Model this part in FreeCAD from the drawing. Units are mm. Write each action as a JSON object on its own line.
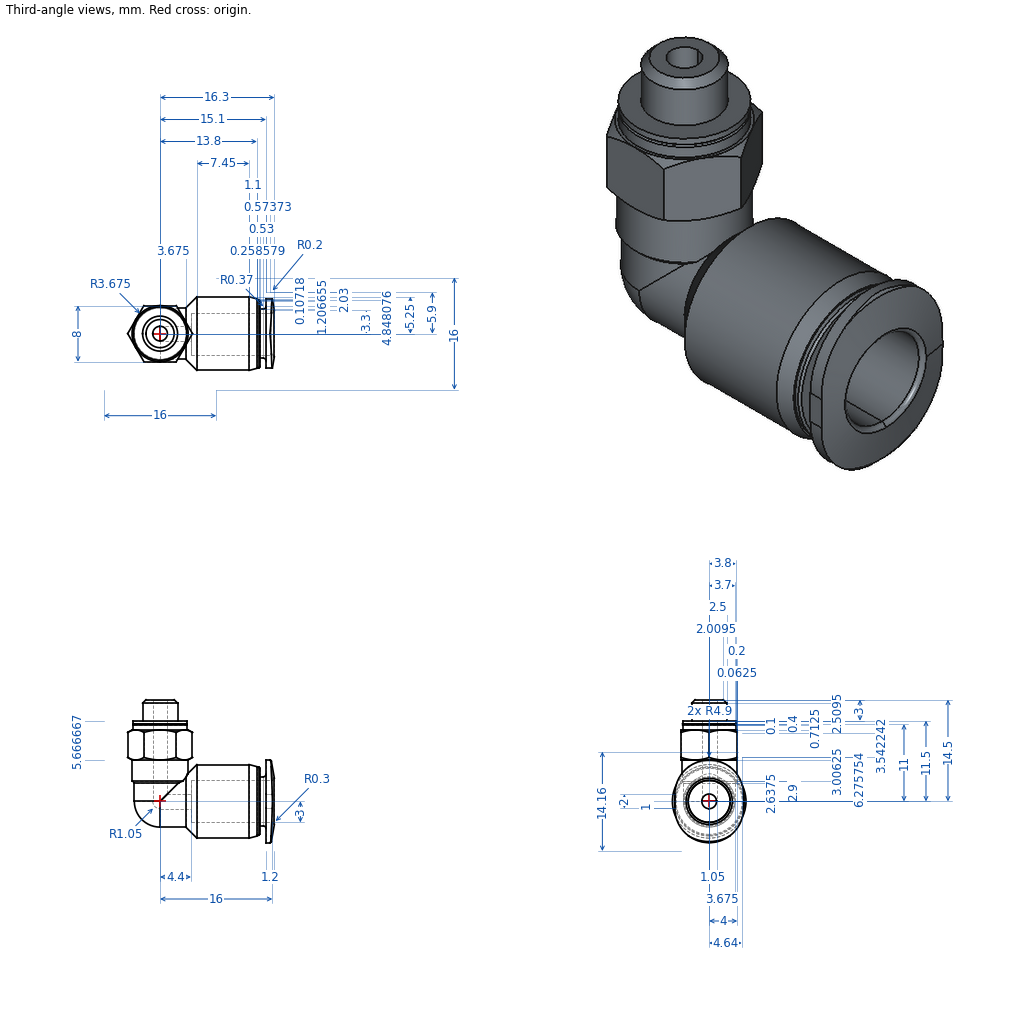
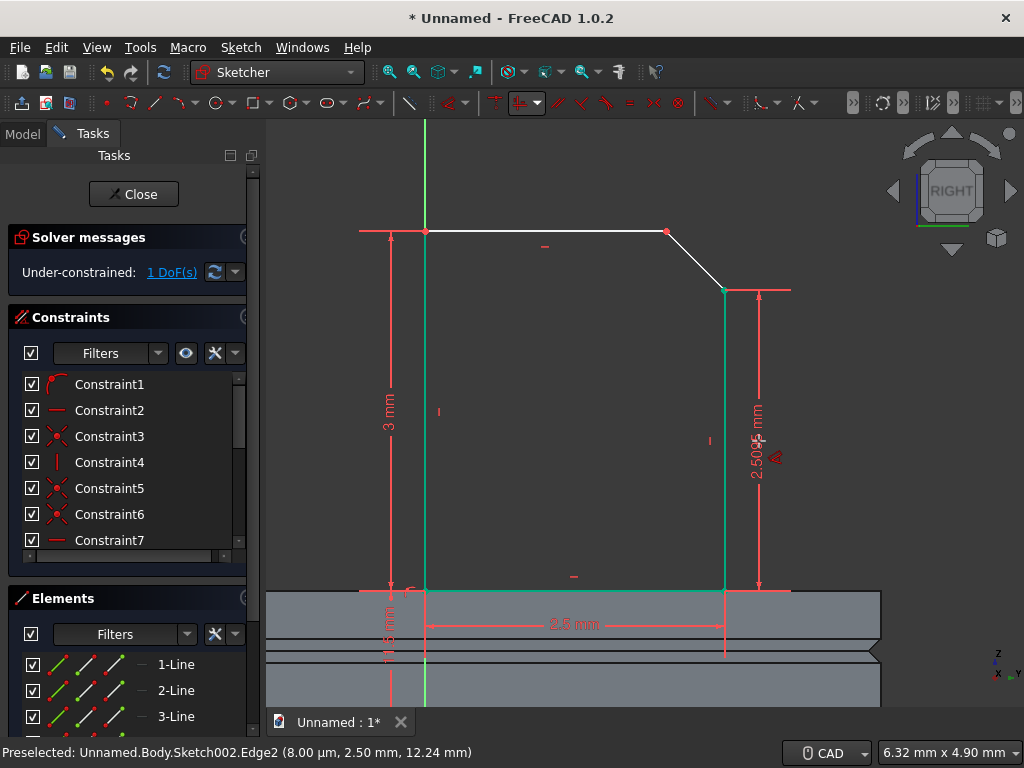
{"action": "left_click", "coordinate": [594, 231]}
{"action": "left_click", "coordinate": [546, 197]}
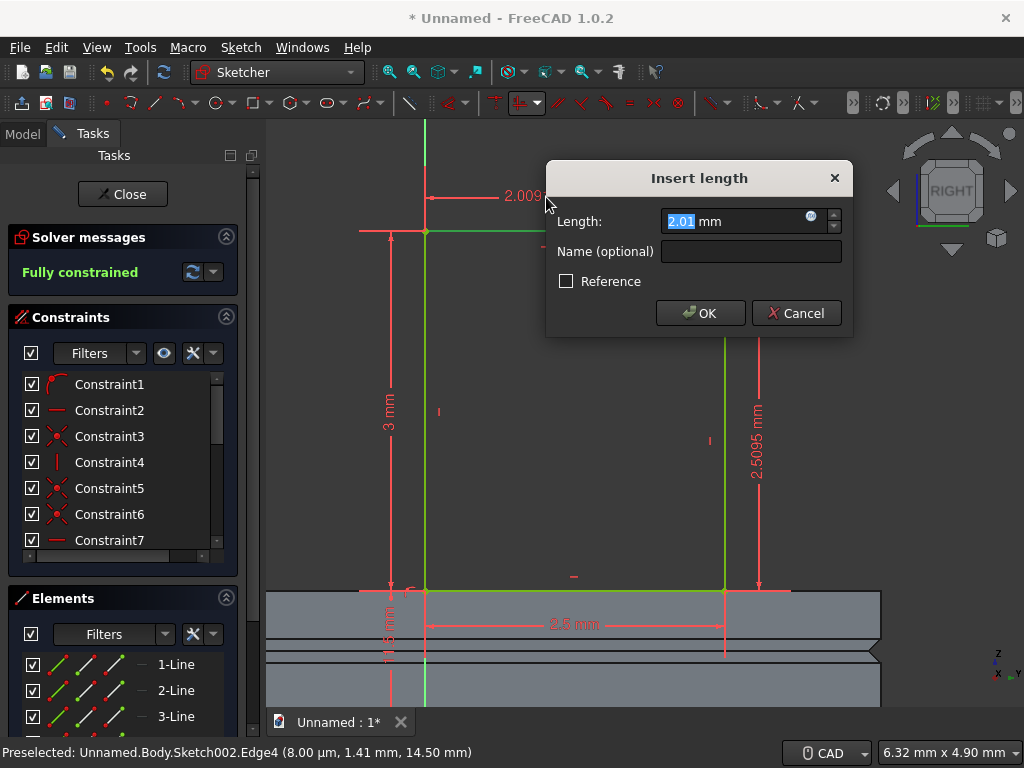
{"action": "type", "text": "2.0095"}
{"action": "key", "text": "Return"}
{"action": "key", "text": "Escape"}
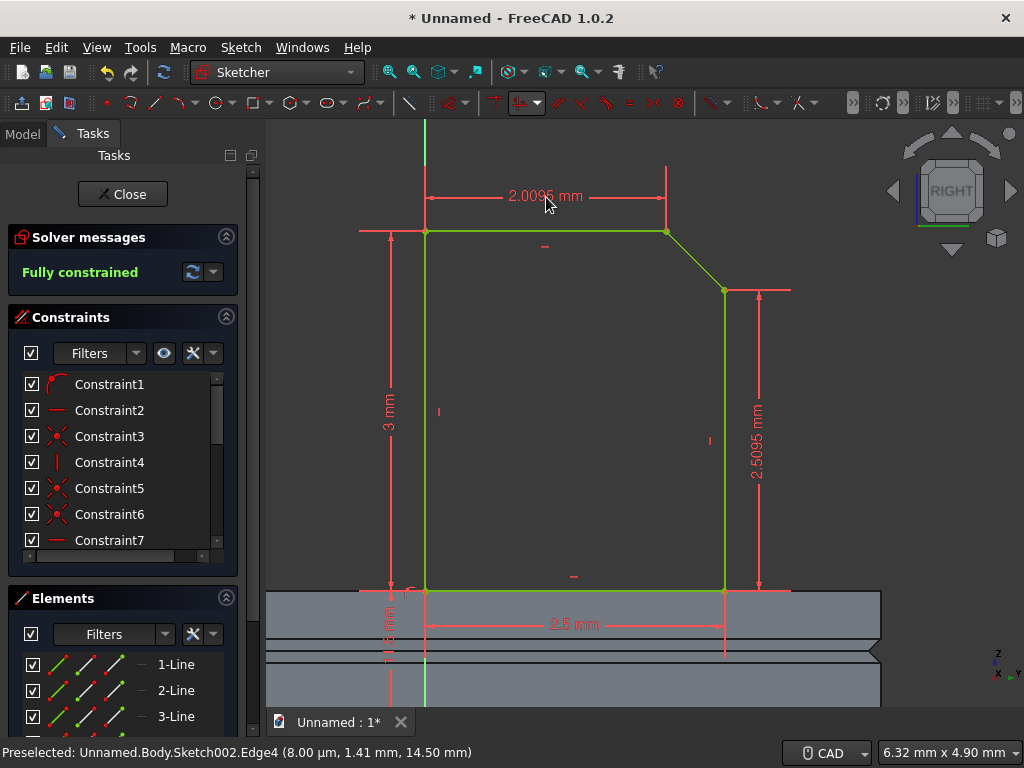
{"action": "left_click", "coordinate": [123, 194]}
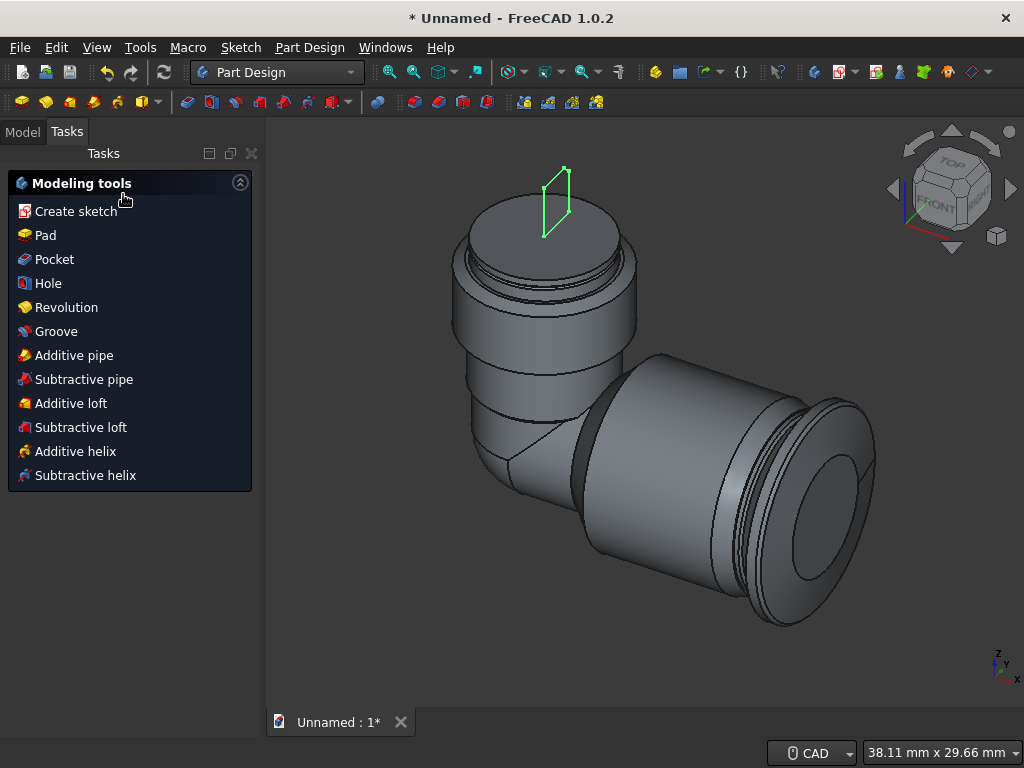
{"action": "left_click", "coordinate": [46, 102]}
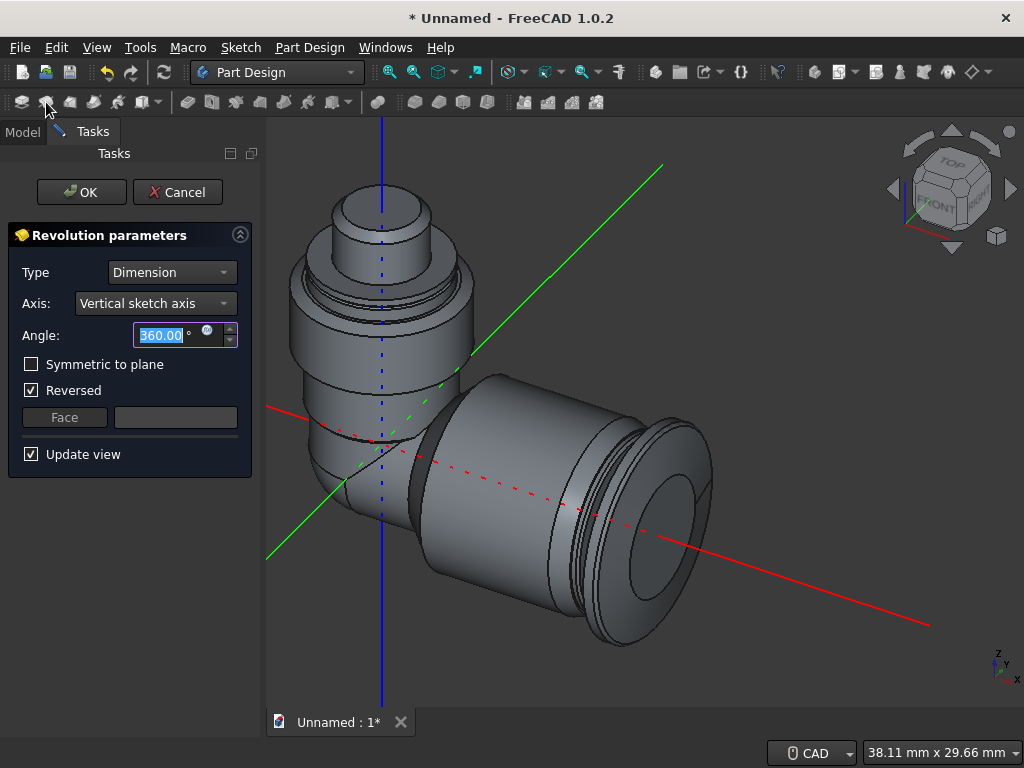
{"action": "left_click", "coordinate": [82, 192]}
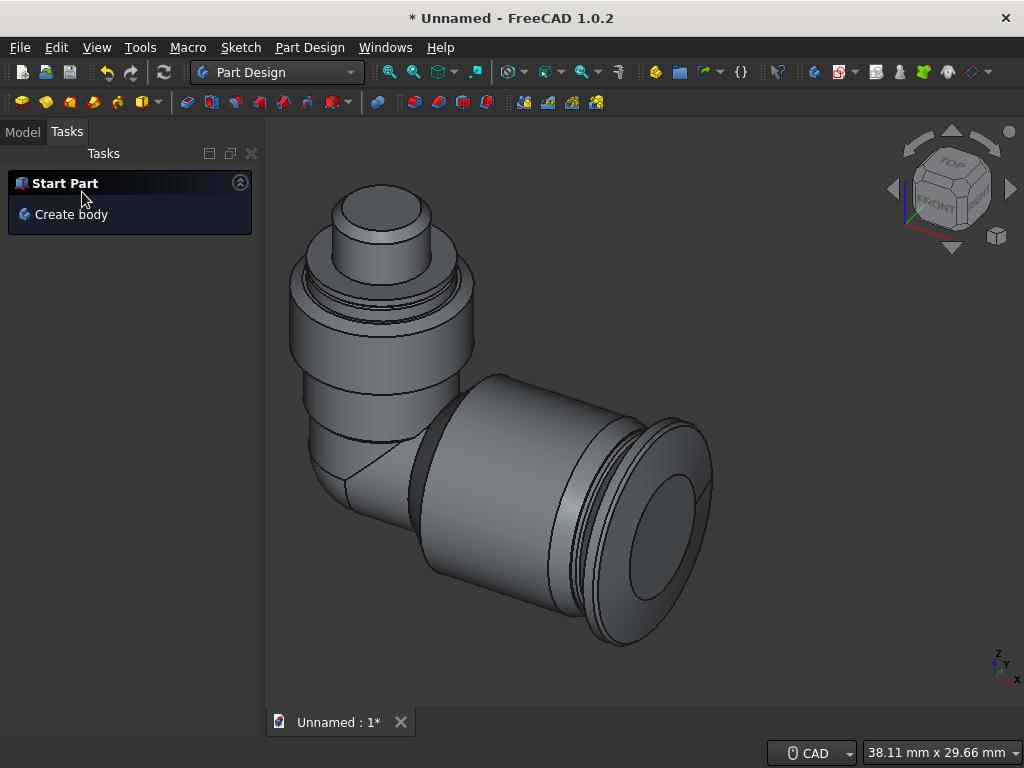
{"action": "left_click", "coordinate": [390, 72]}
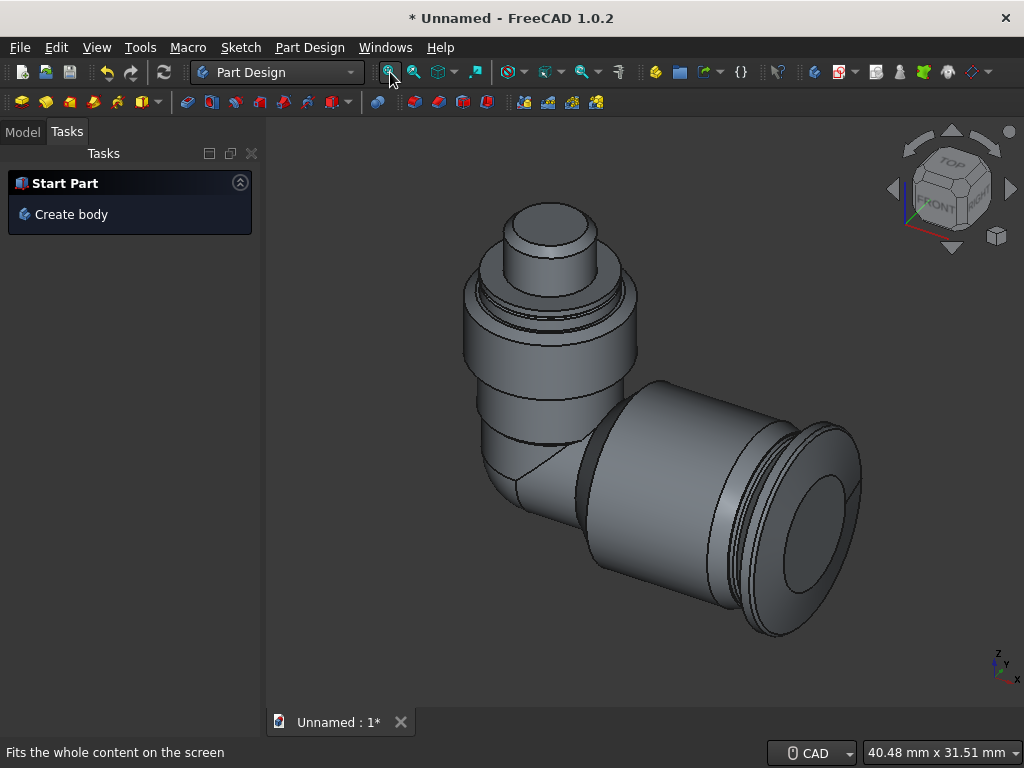
{"action": "left_click", "coordinate": [815, 533]}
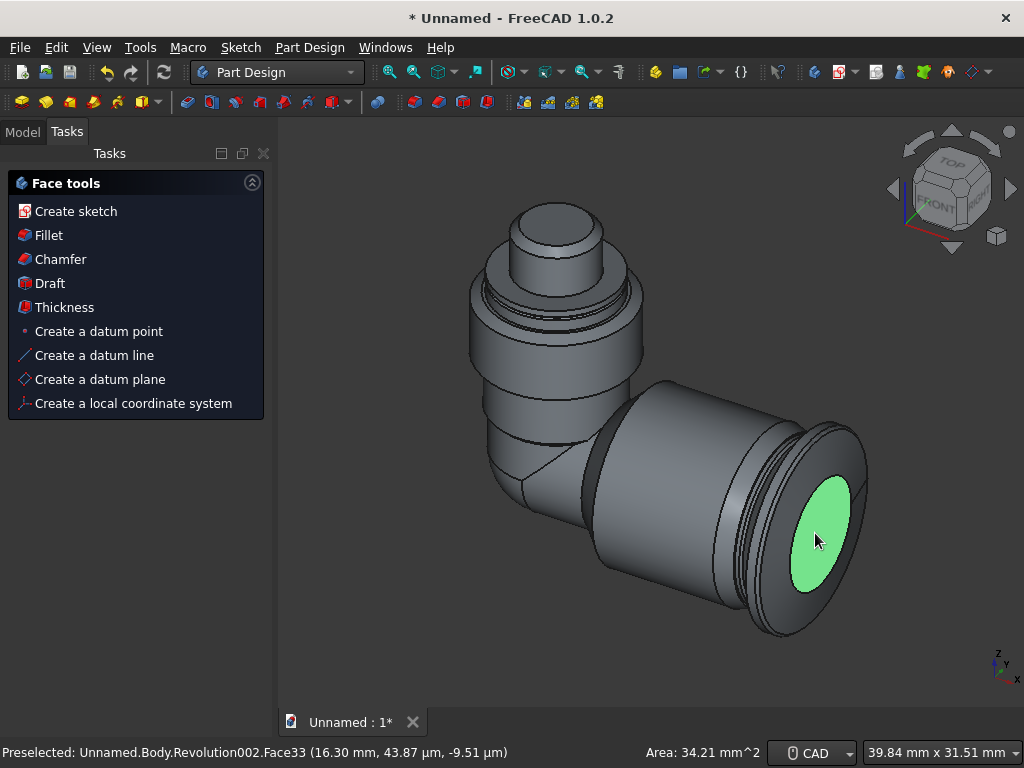
{"action": "left_click", "coordinate": [840, 72]}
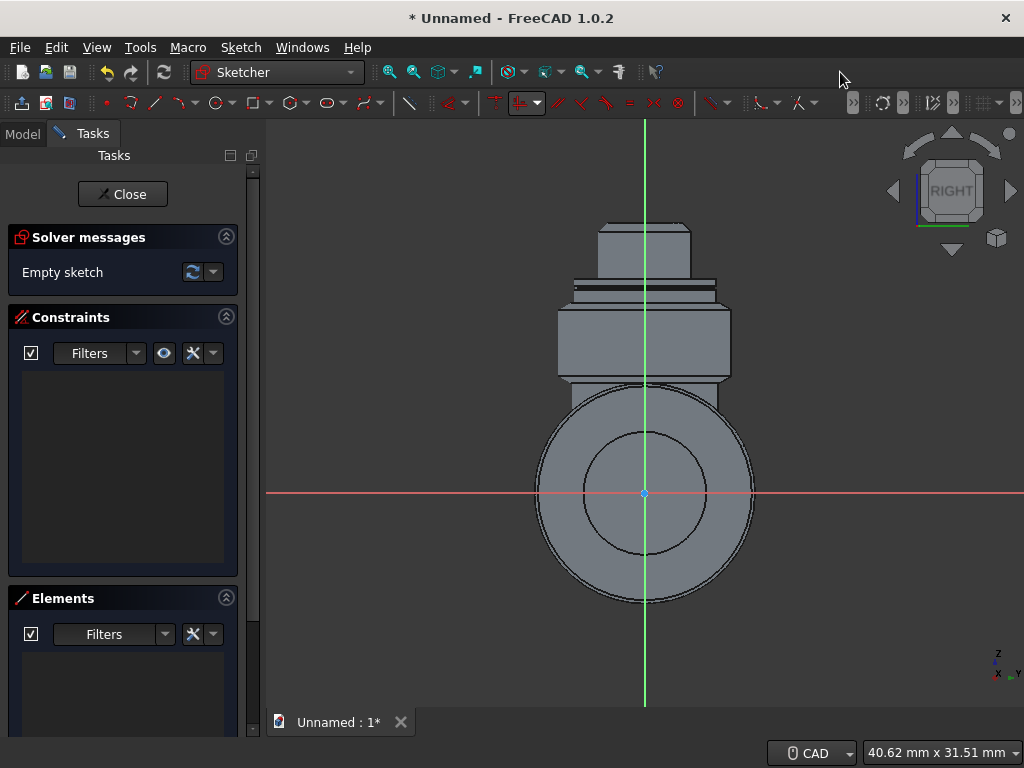
{"action": "left_click", "coordinate": [290, 104]}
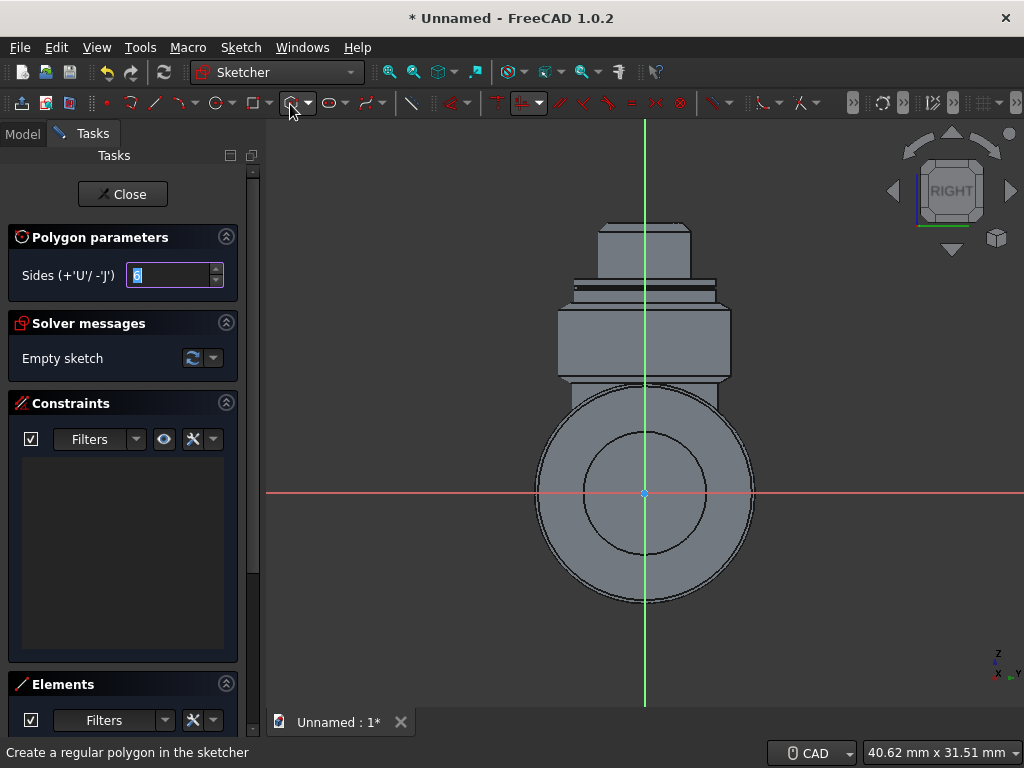
{"action": "left_click", "coordinate": [645, 493]}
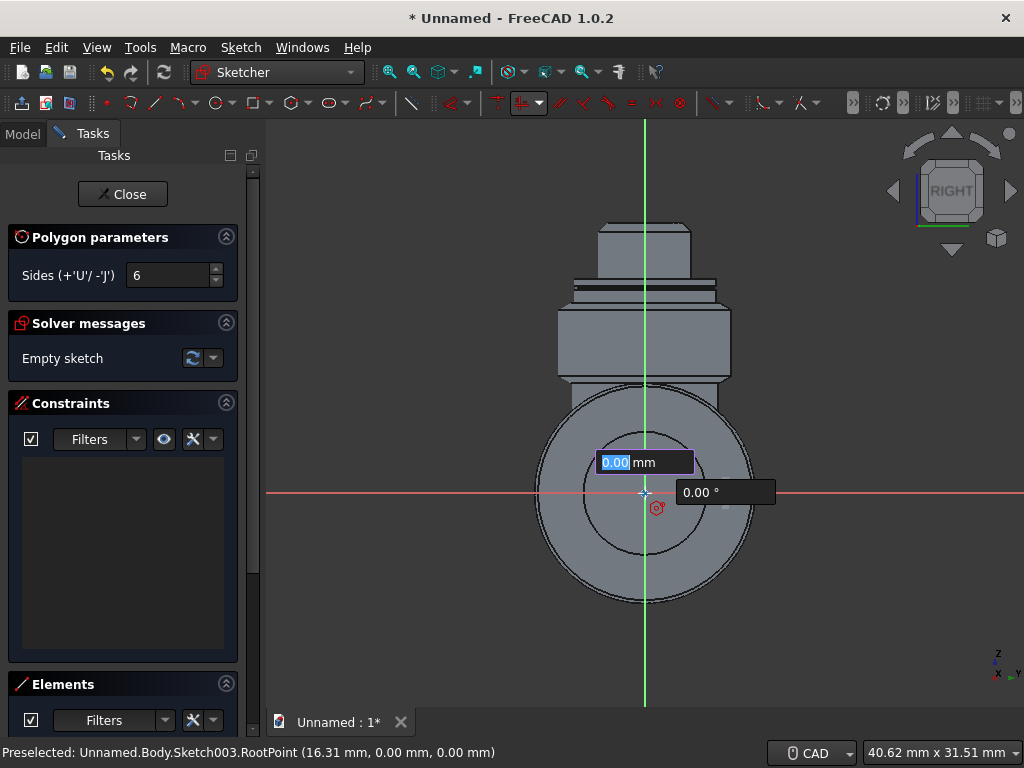
{"action": "left_click", "coordinate": [492, 493]}
{"action": "right_click", "coordinate": [492, 493]}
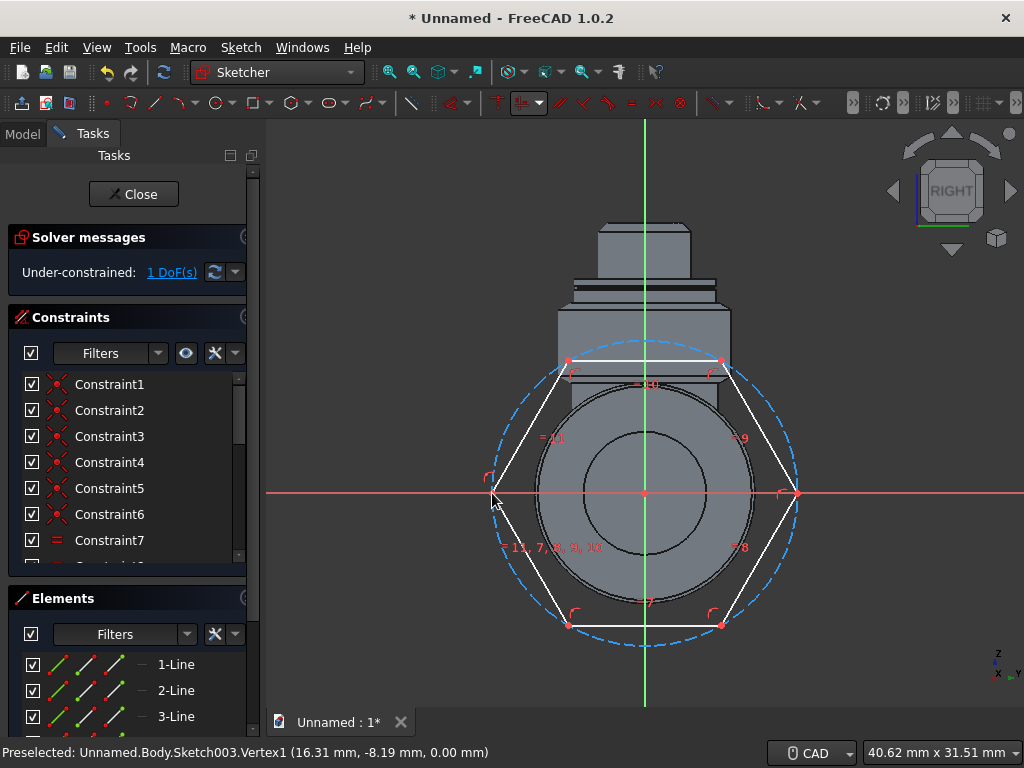
{"action": "left_click", "coordinate": [330, 104]}